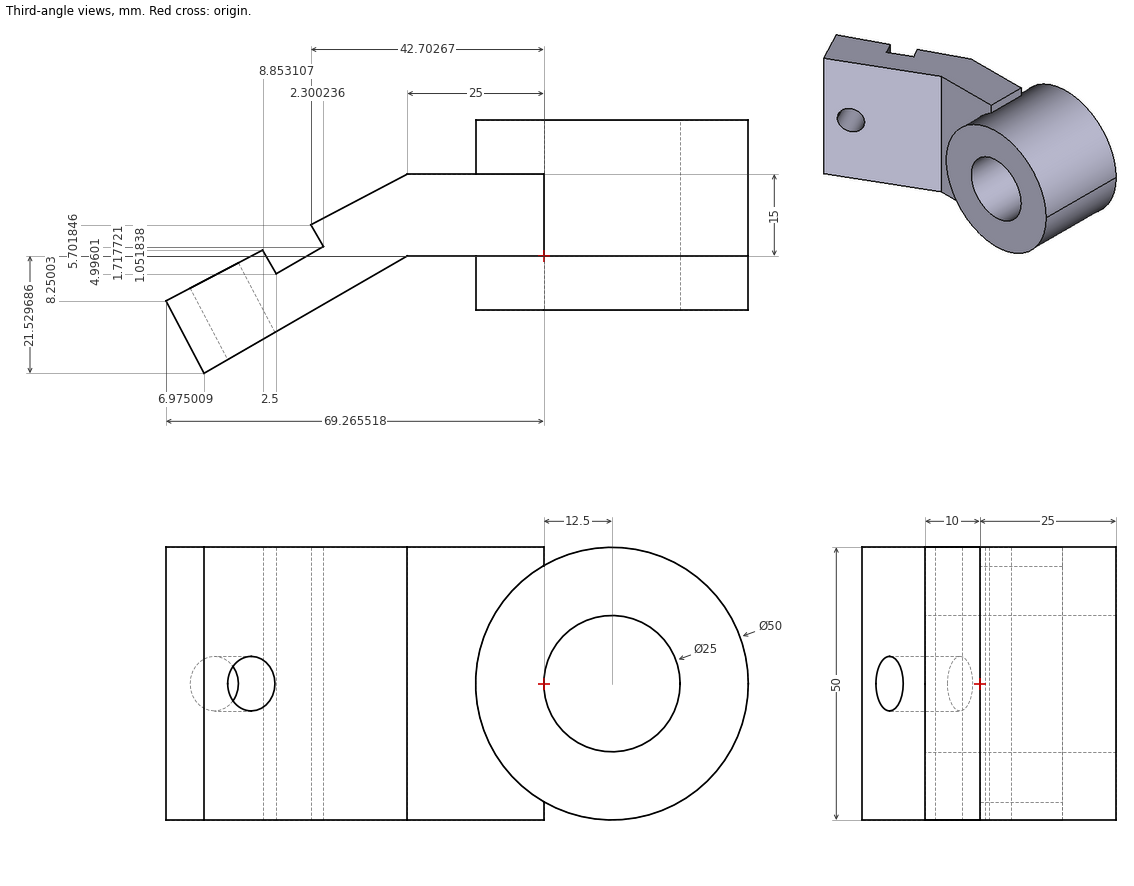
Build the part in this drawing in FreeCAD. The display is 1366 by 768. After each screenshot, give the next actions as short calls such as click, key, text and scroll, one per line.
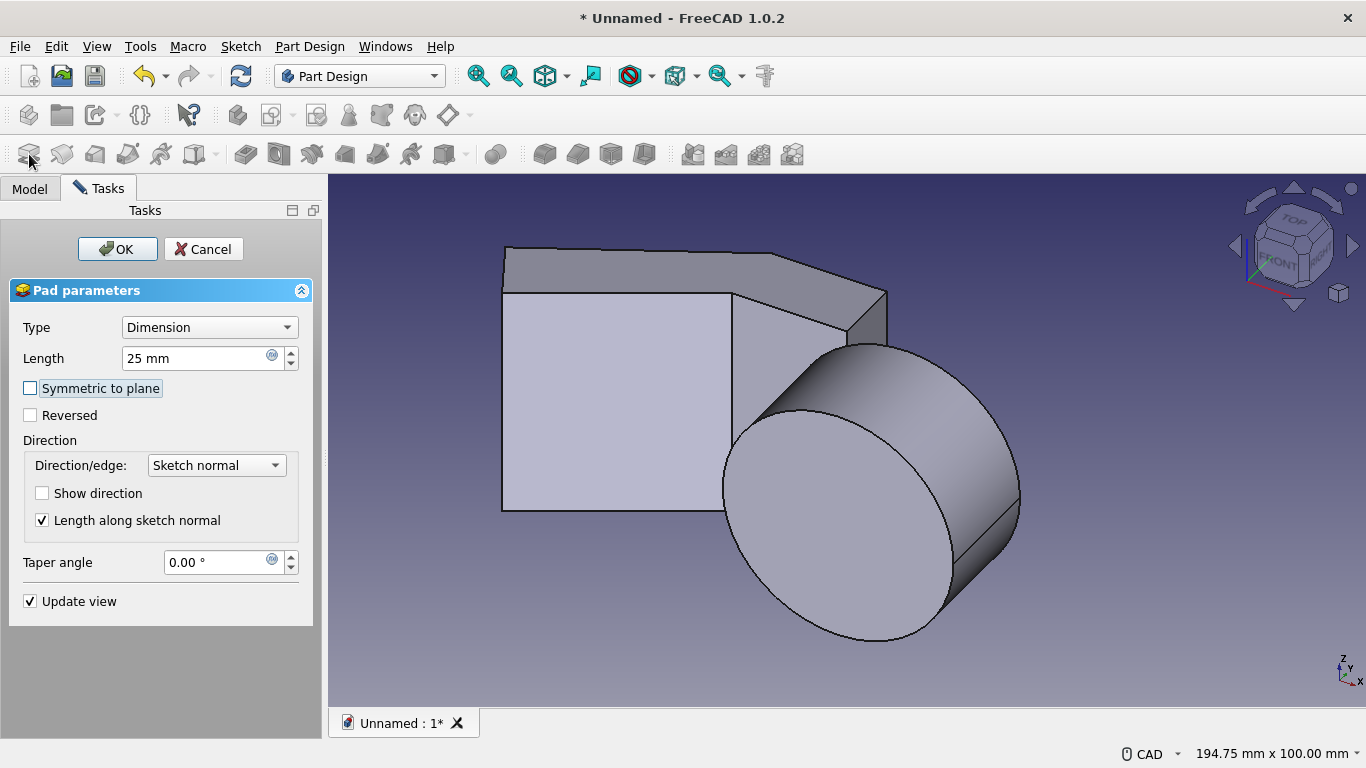
click(31, 415)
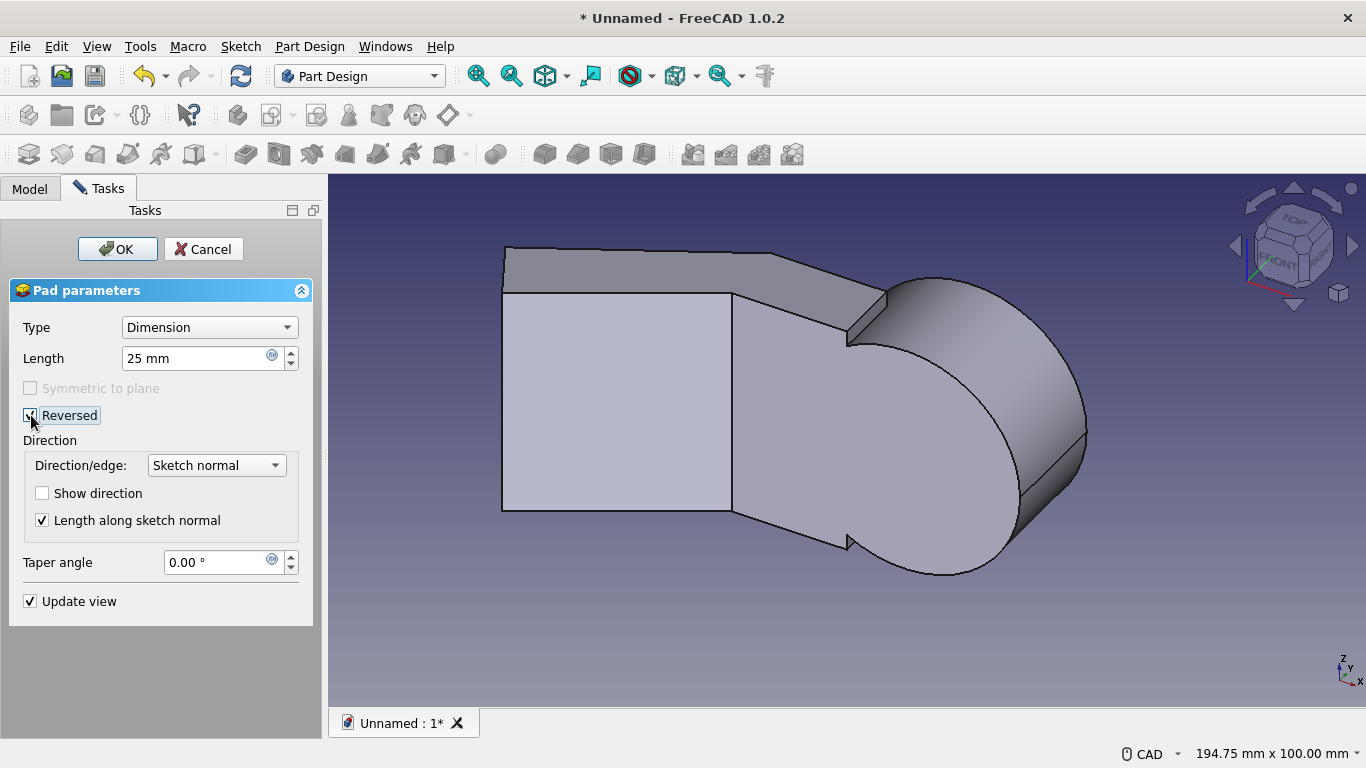
click(118, 249)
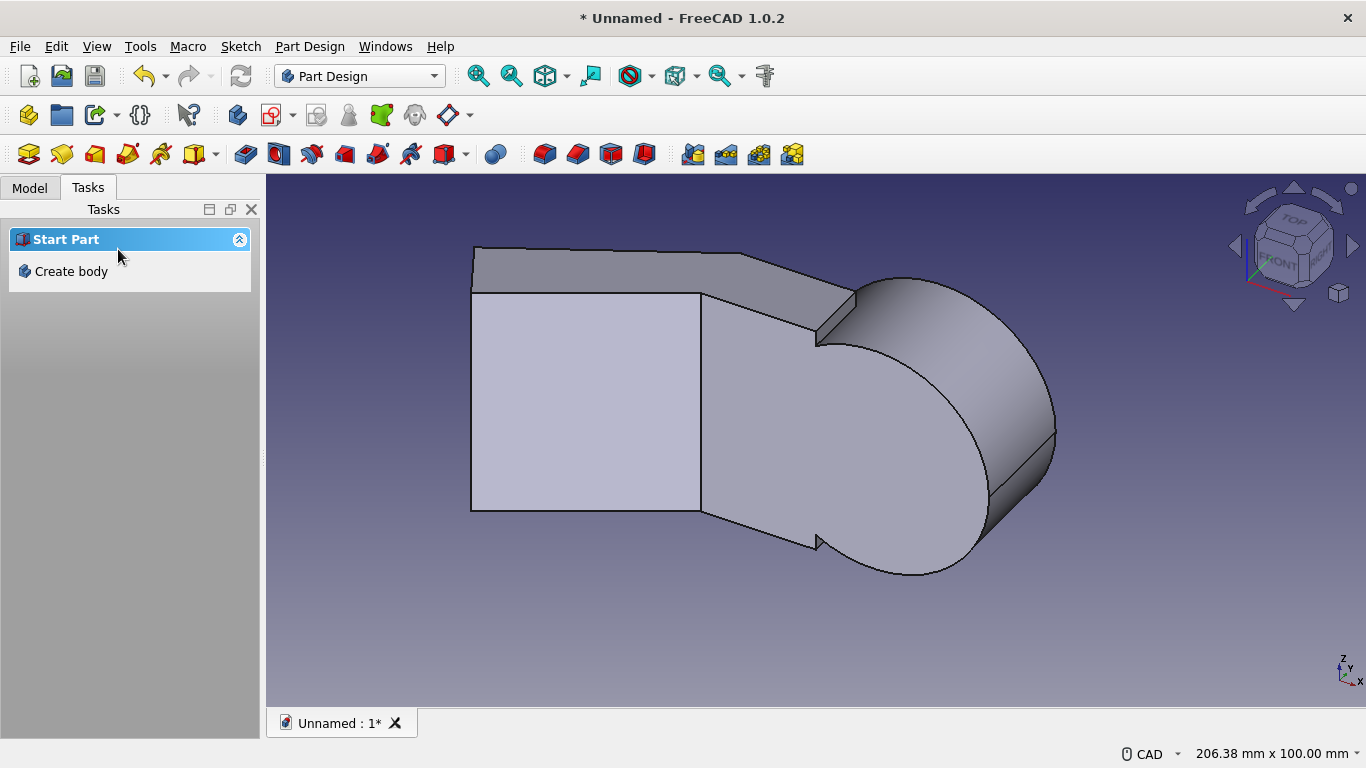
click(479, 76)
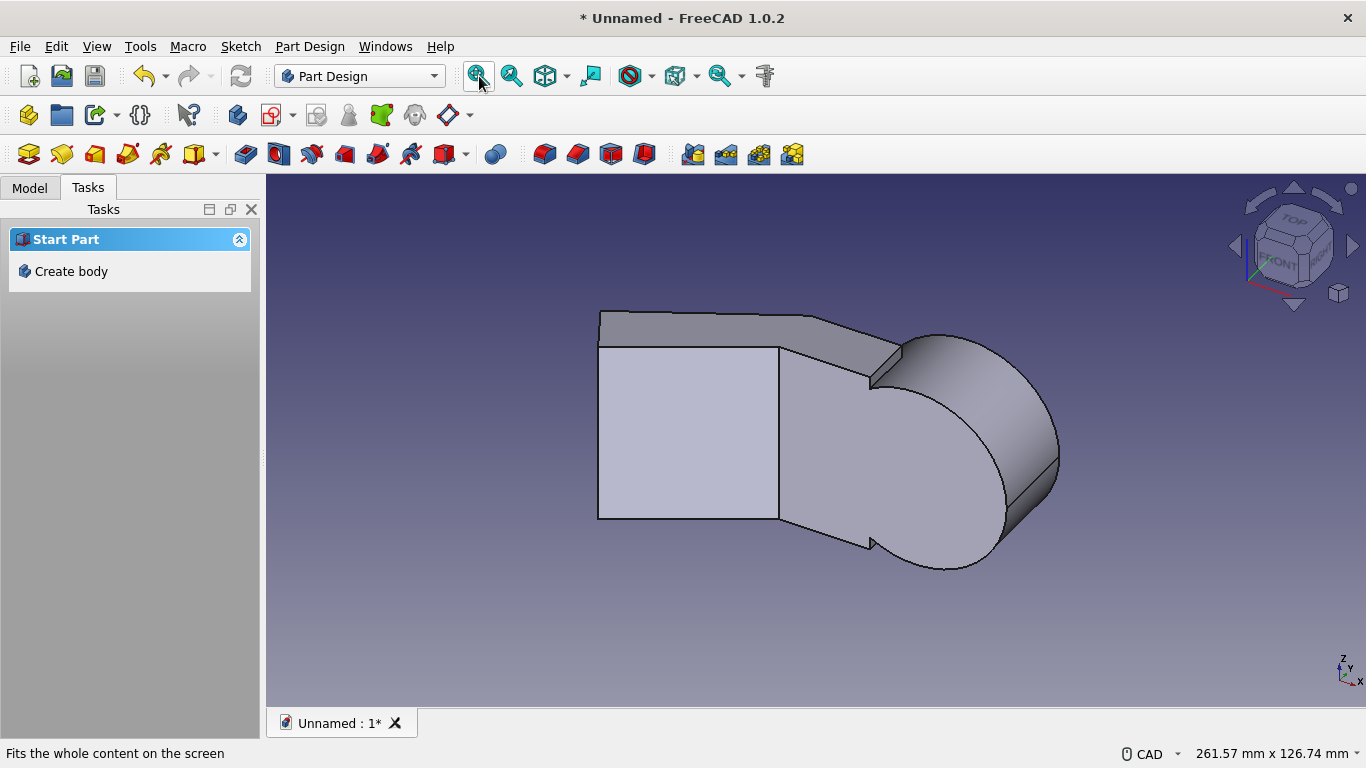
click(30, 188)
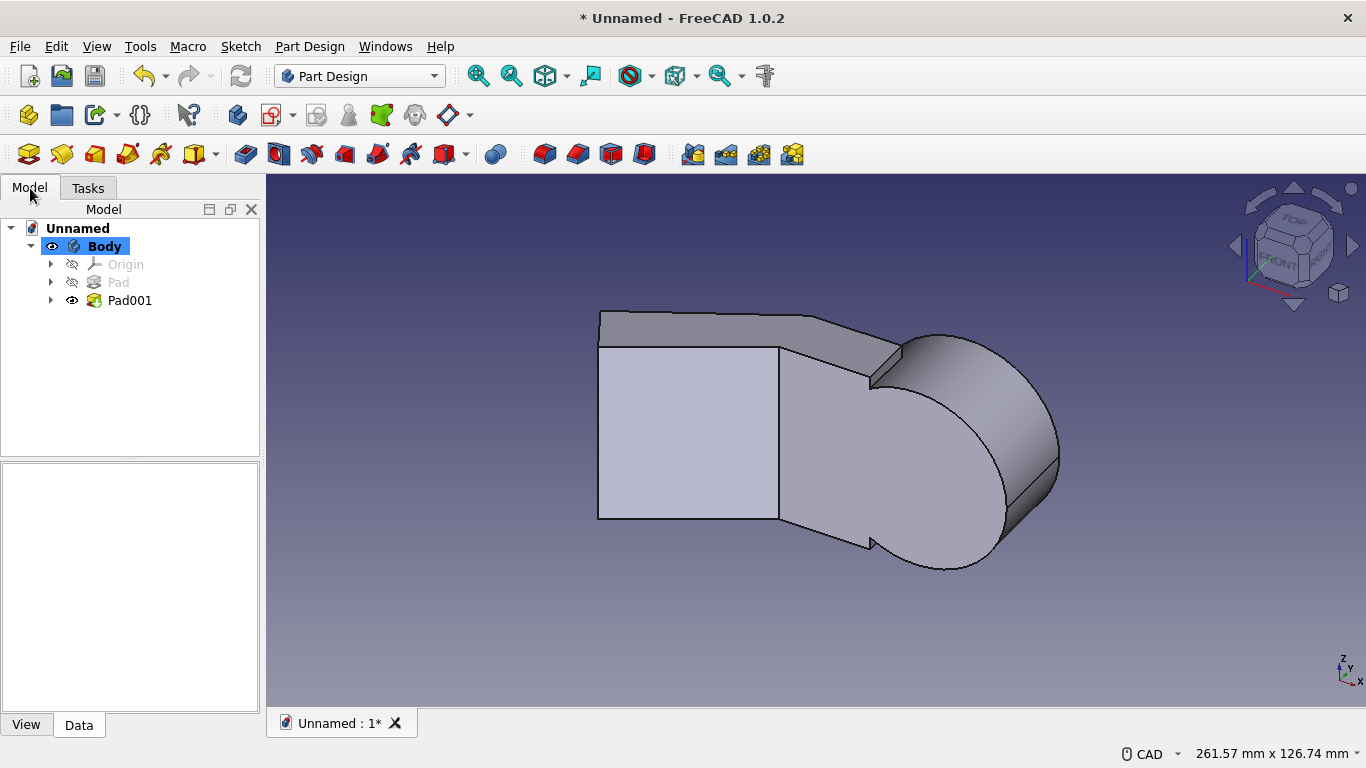
click(51, 264)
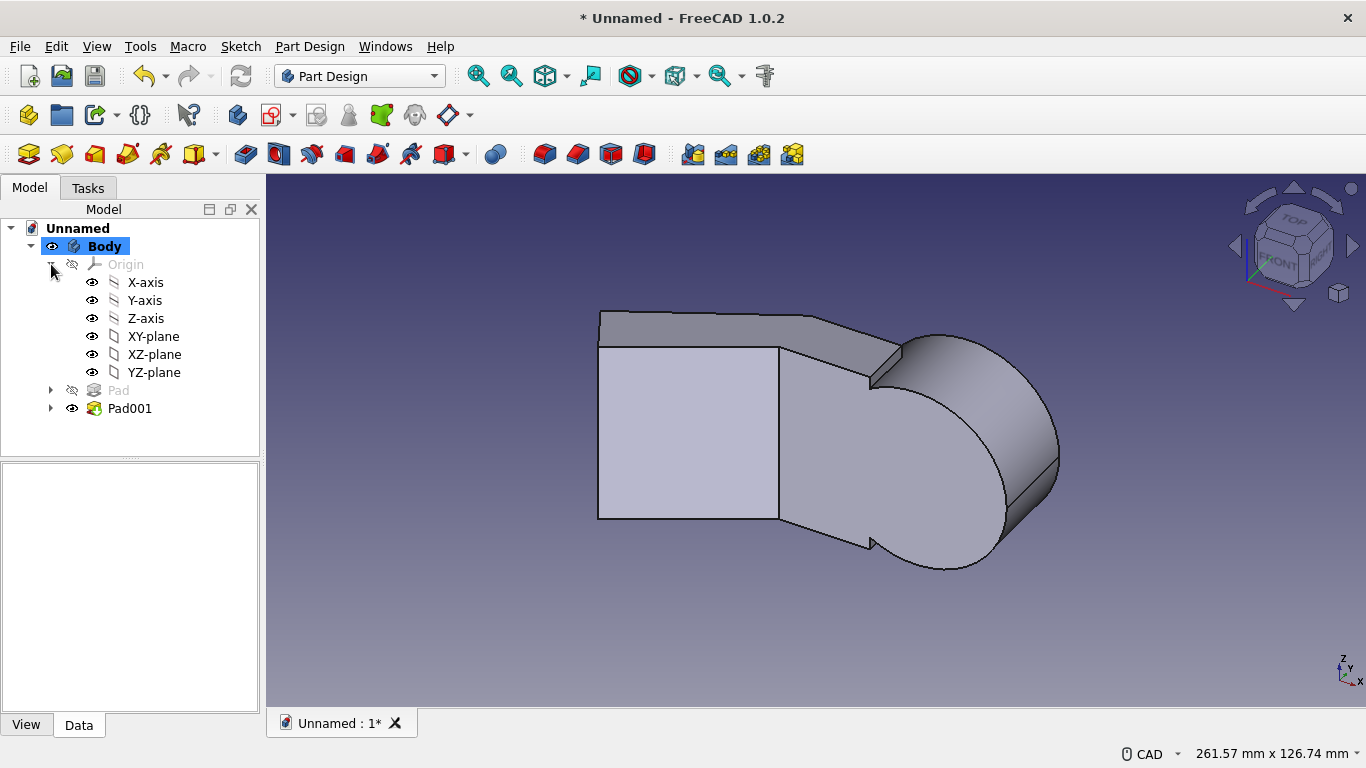
click(137, 354)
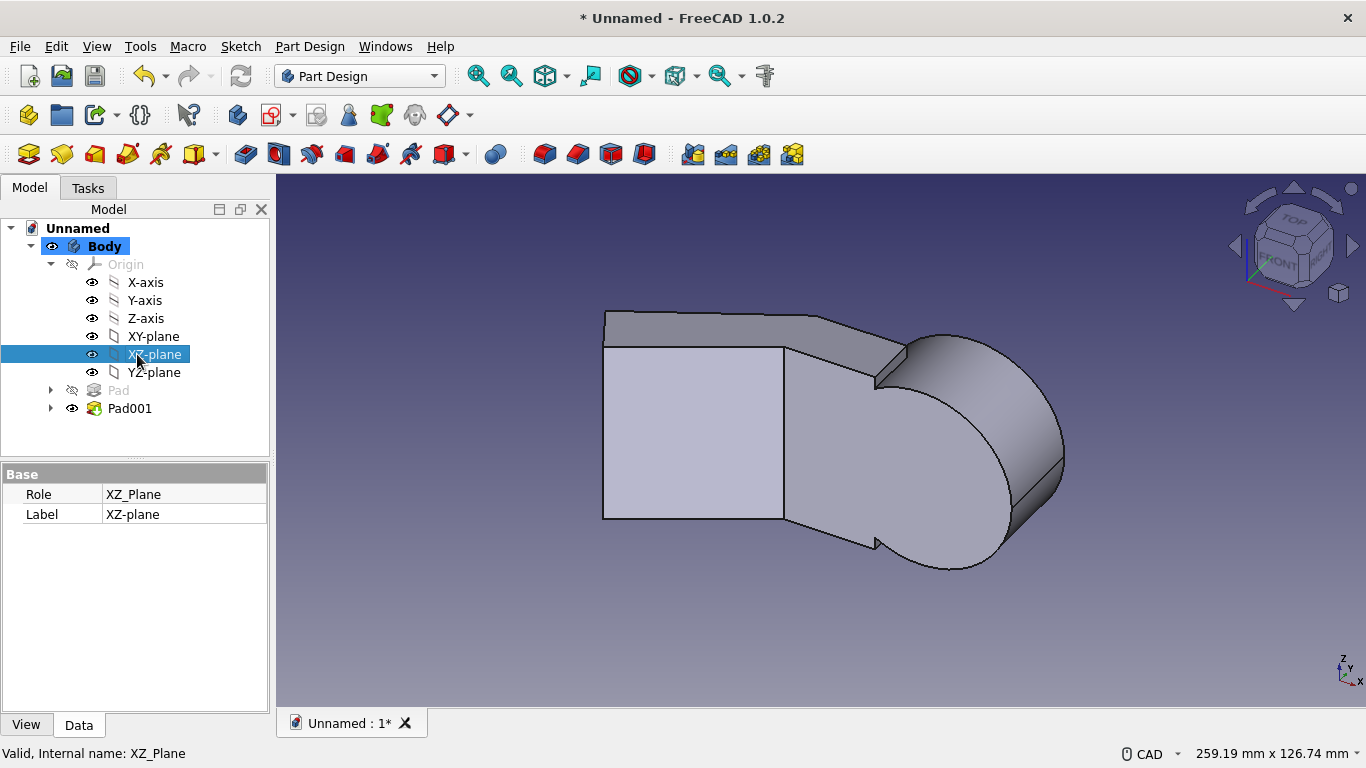
click(448, 116)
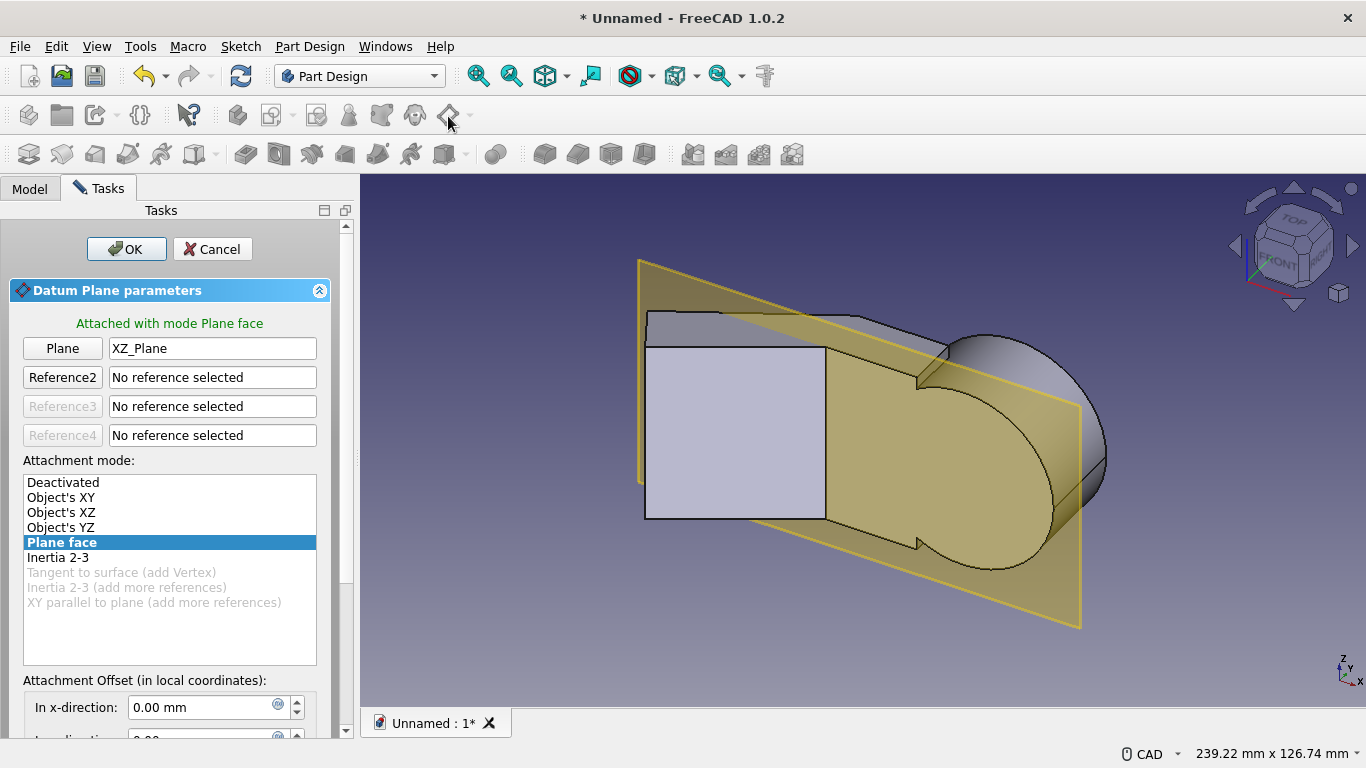
scroll(346, 479, down, 2)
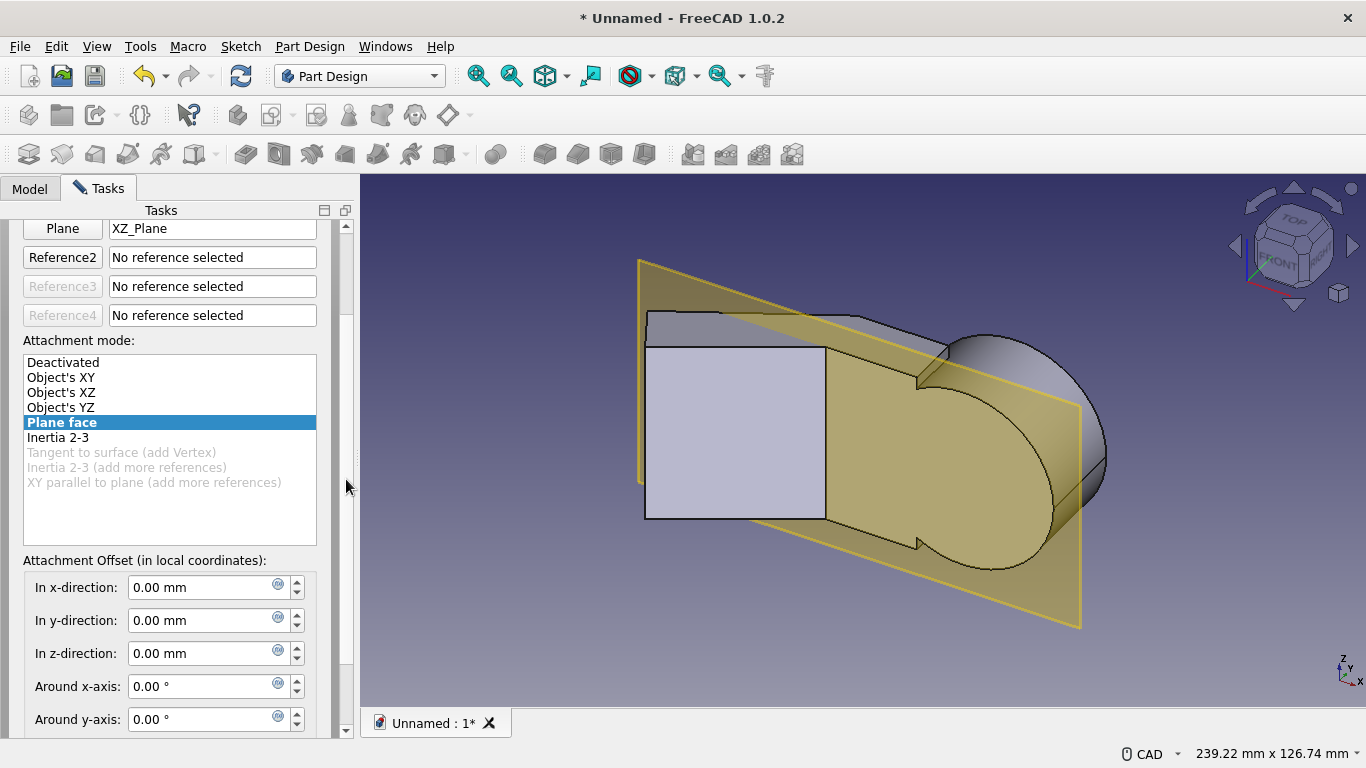
triple_click(210, 654)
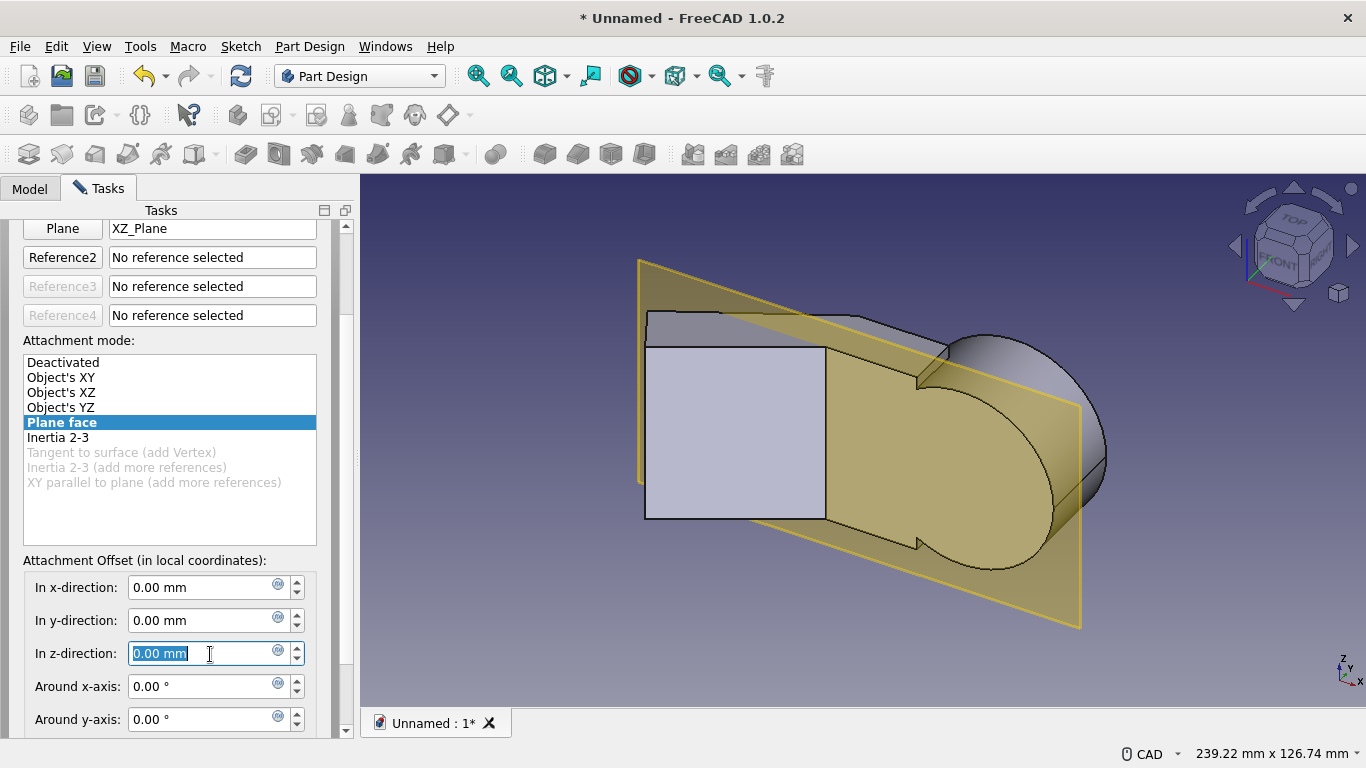
text(10)
key(Tab)